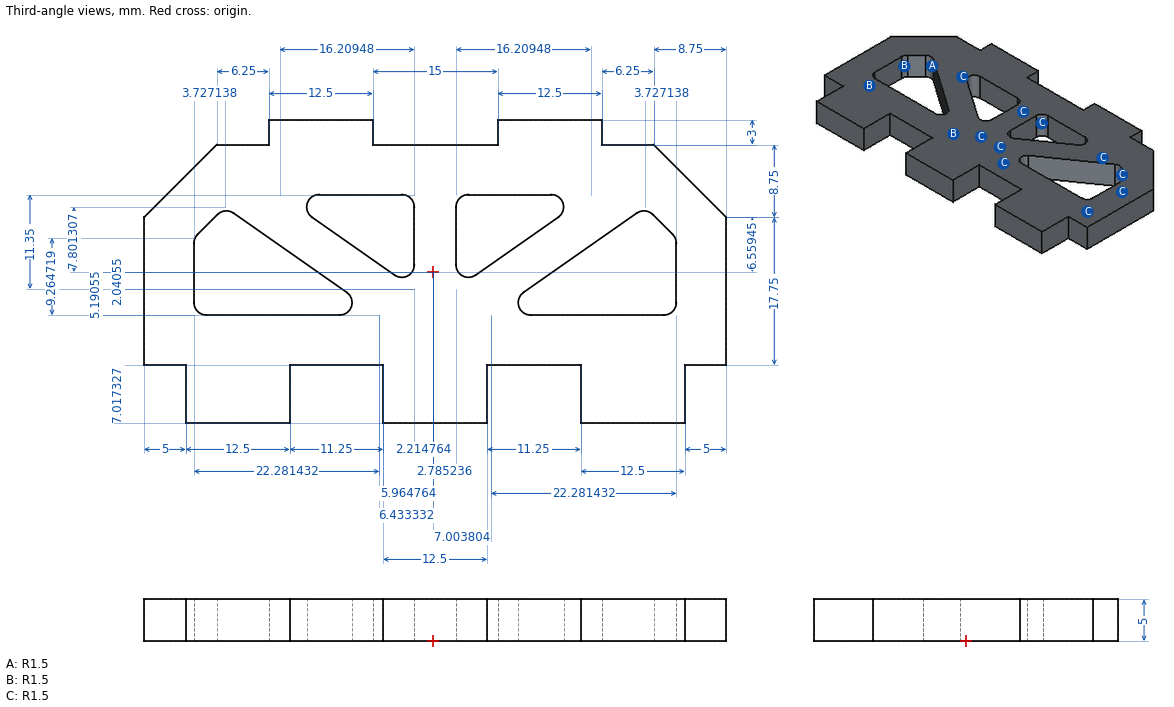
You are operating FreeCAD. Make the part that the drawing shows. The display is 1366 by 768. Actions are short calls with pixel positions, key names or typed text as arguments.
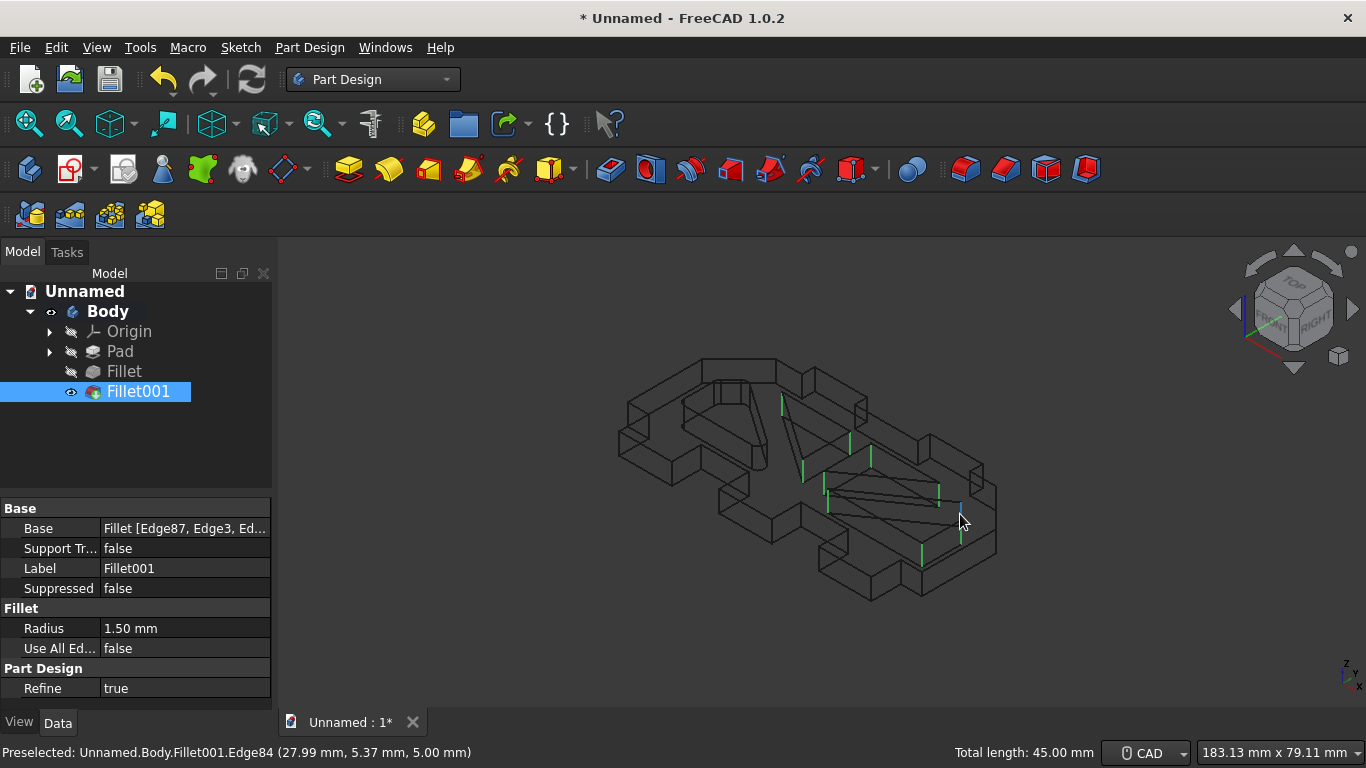
key(2)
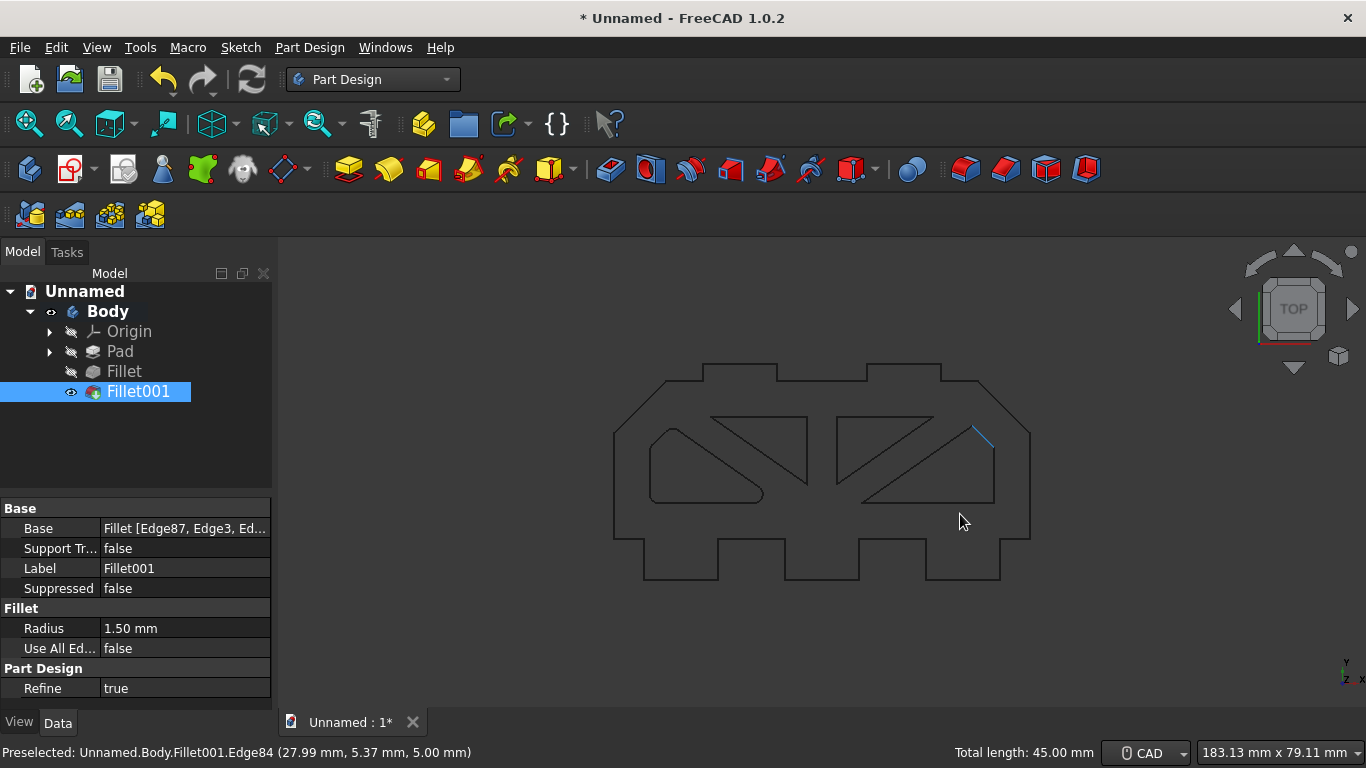
scroll(972, 425, up, 6)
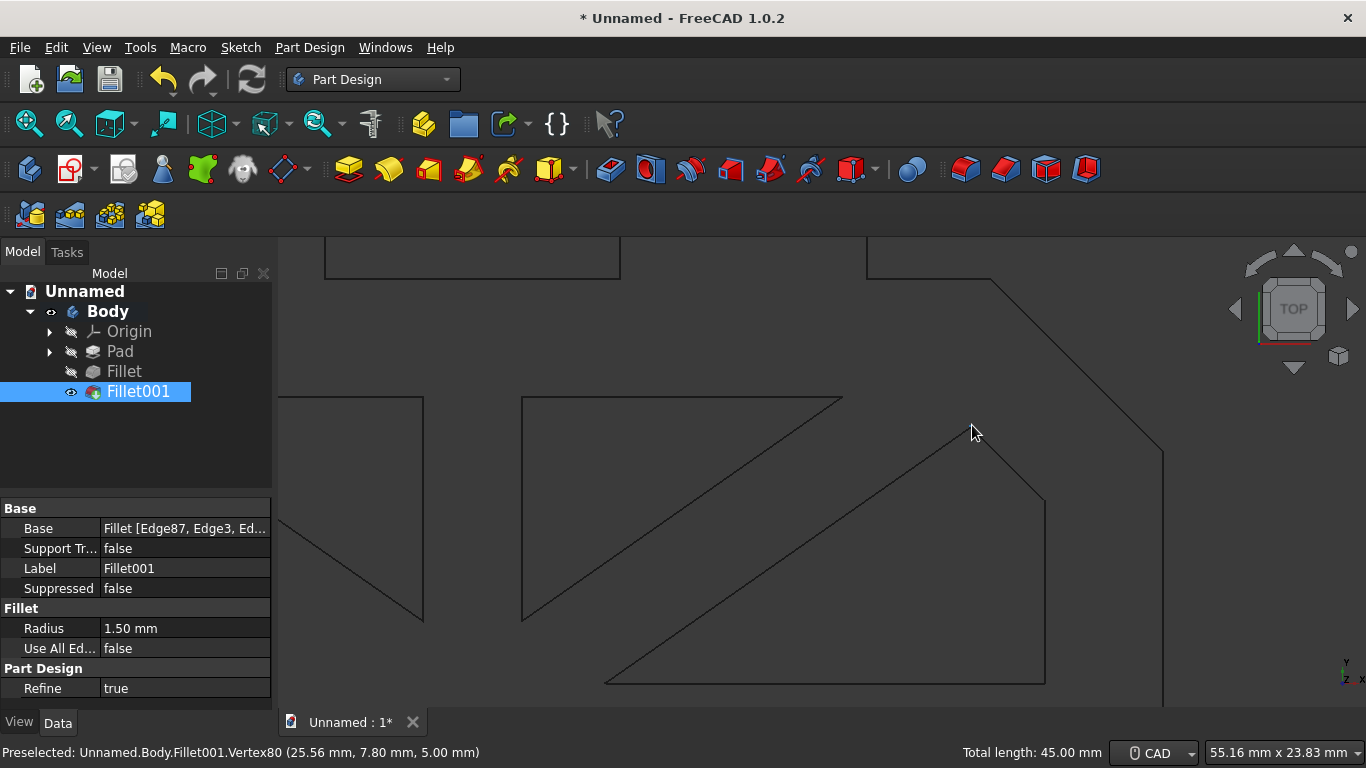
key(v)
key(f)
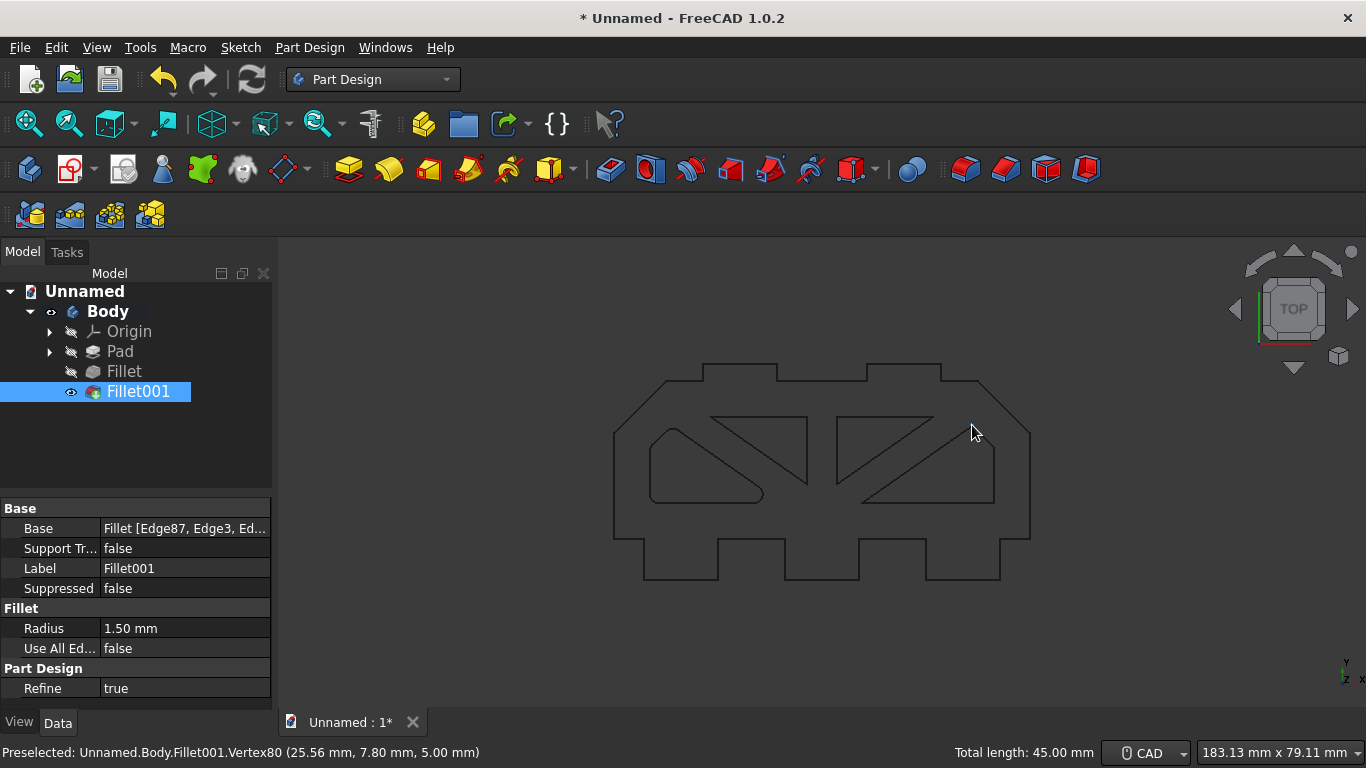
key(1)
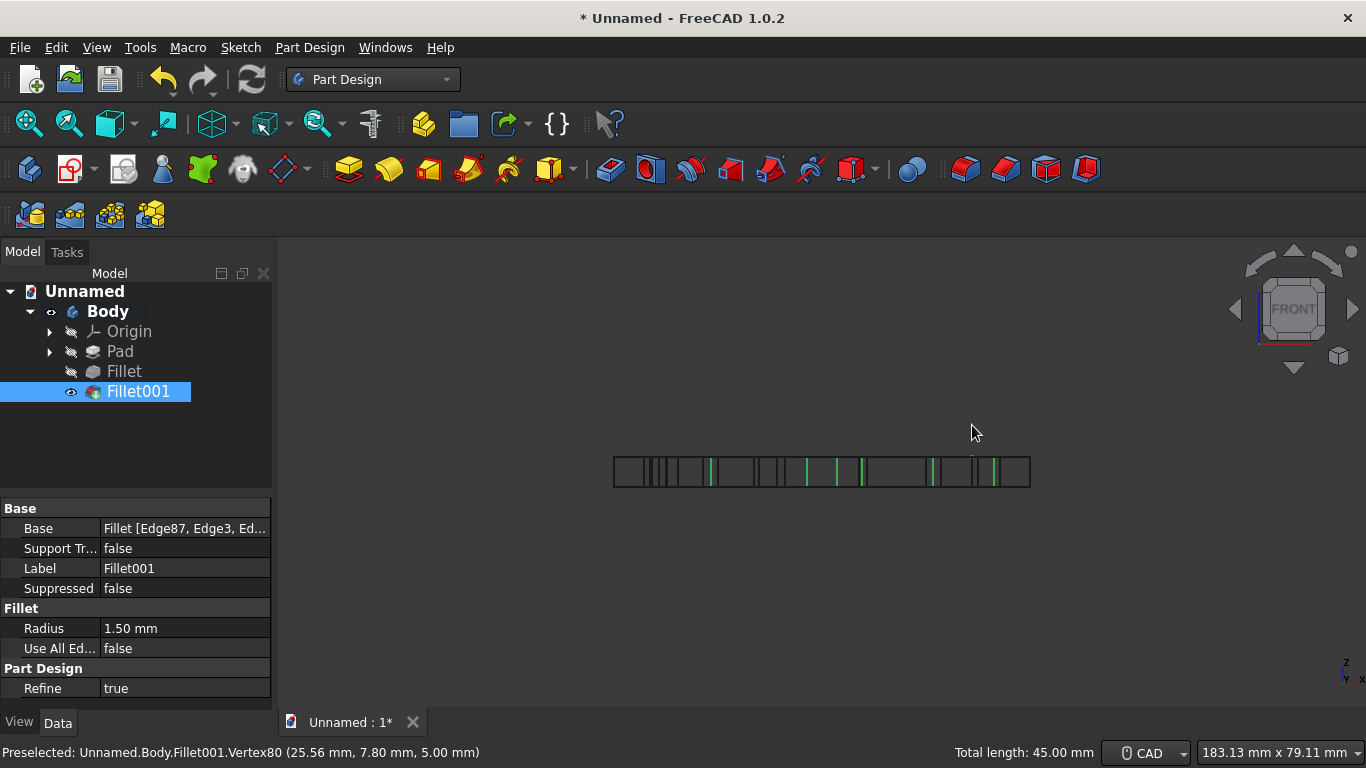
key(v)
key(f)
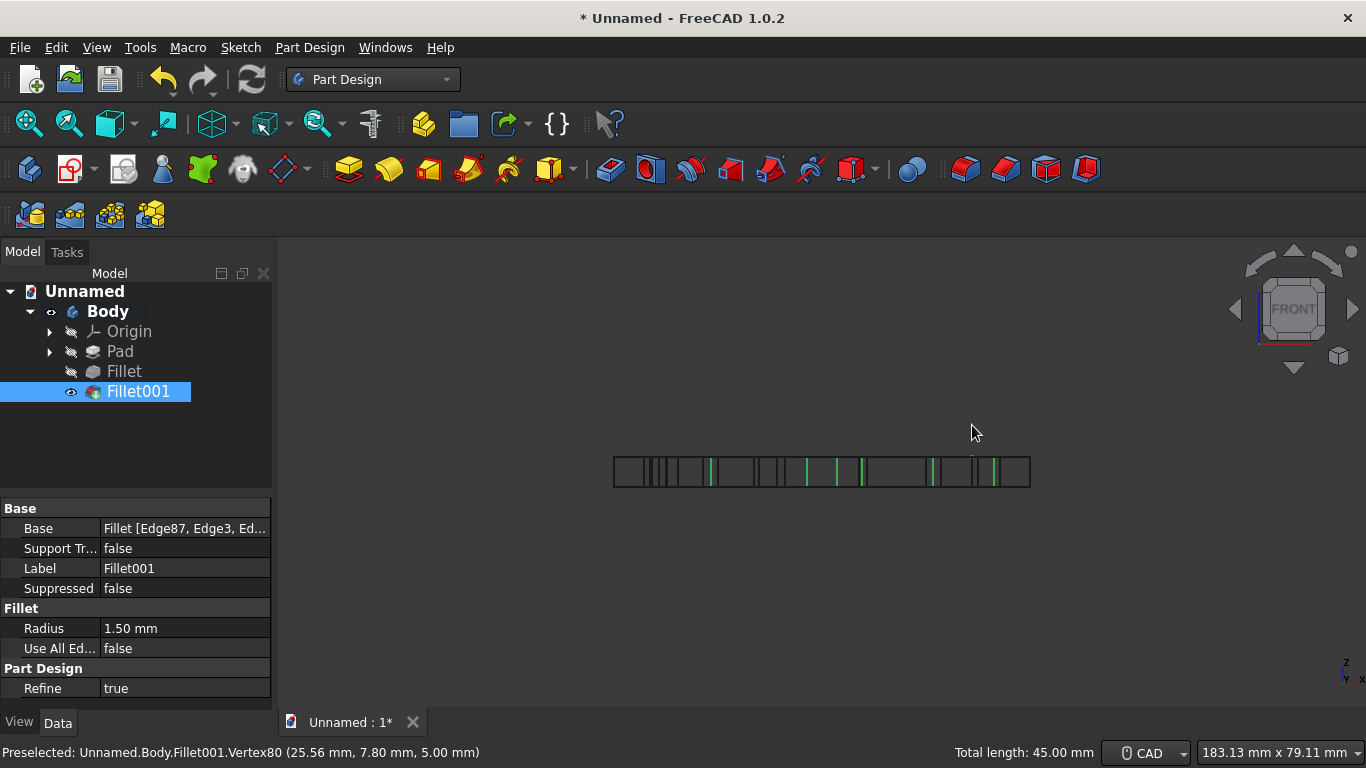
click(972, 471, ctrl)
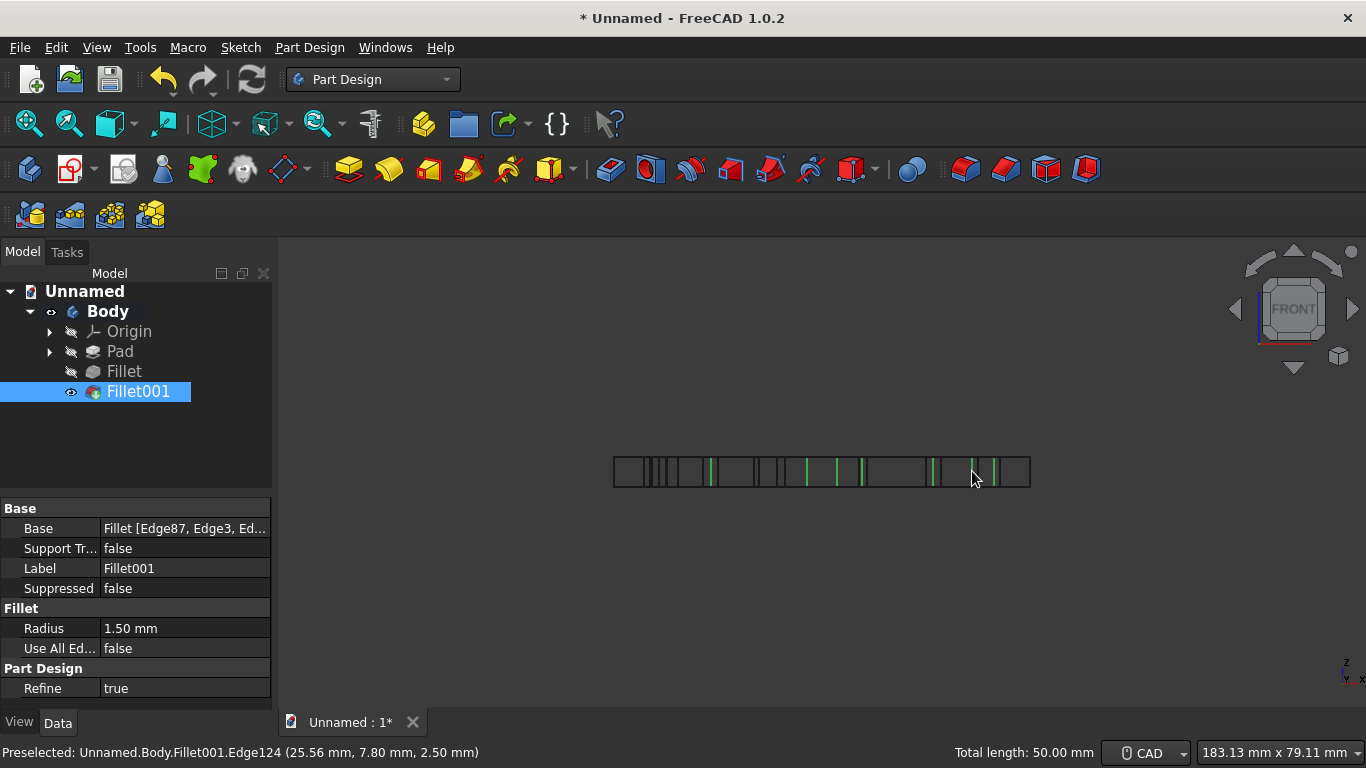
key(v)
key(1)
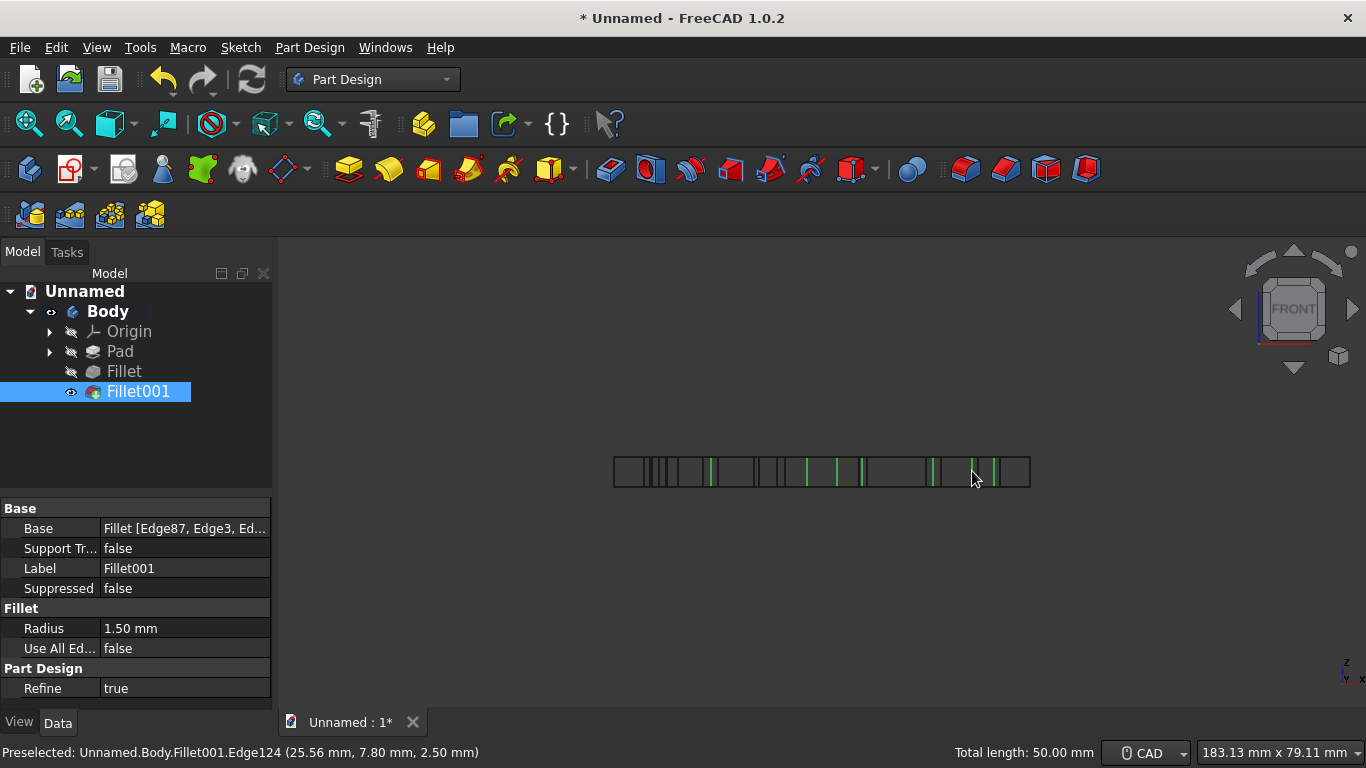
click(966, 170)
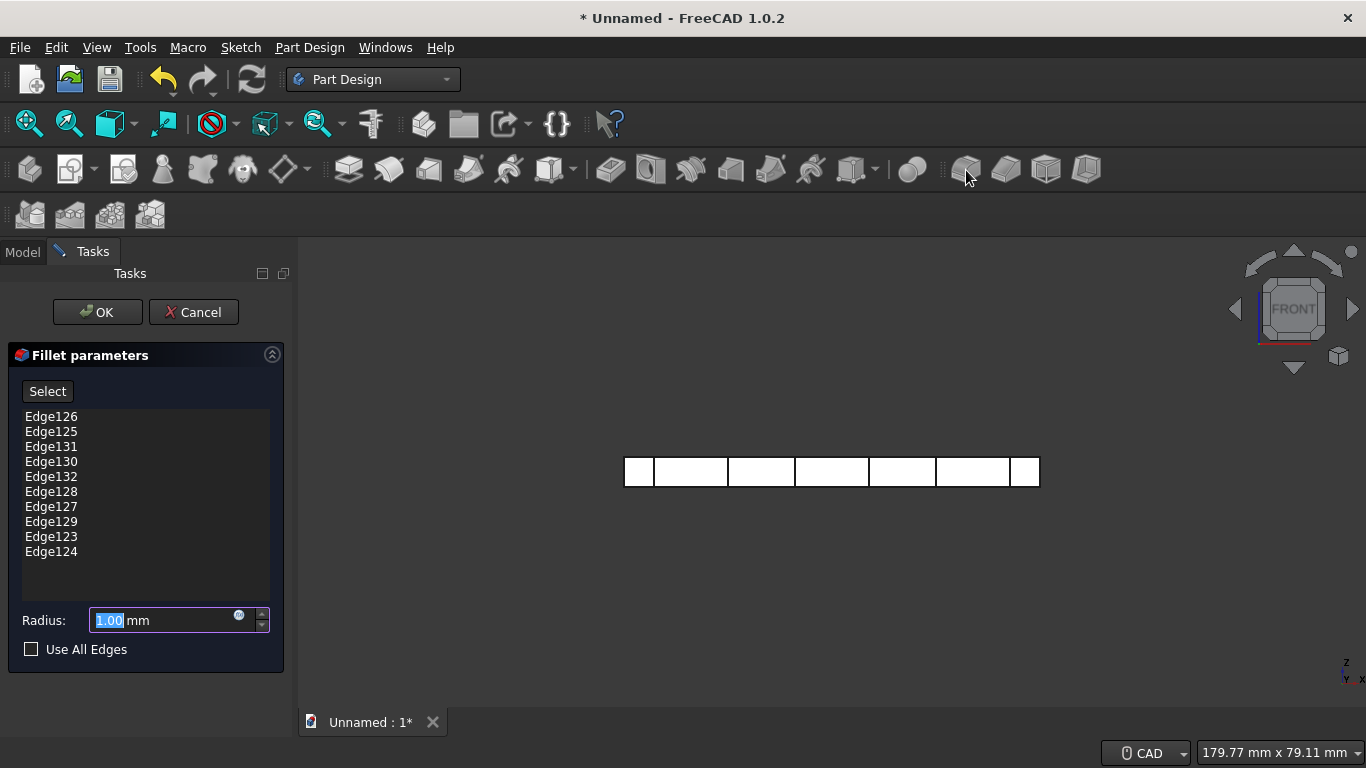
text(1.5)
key(Tab)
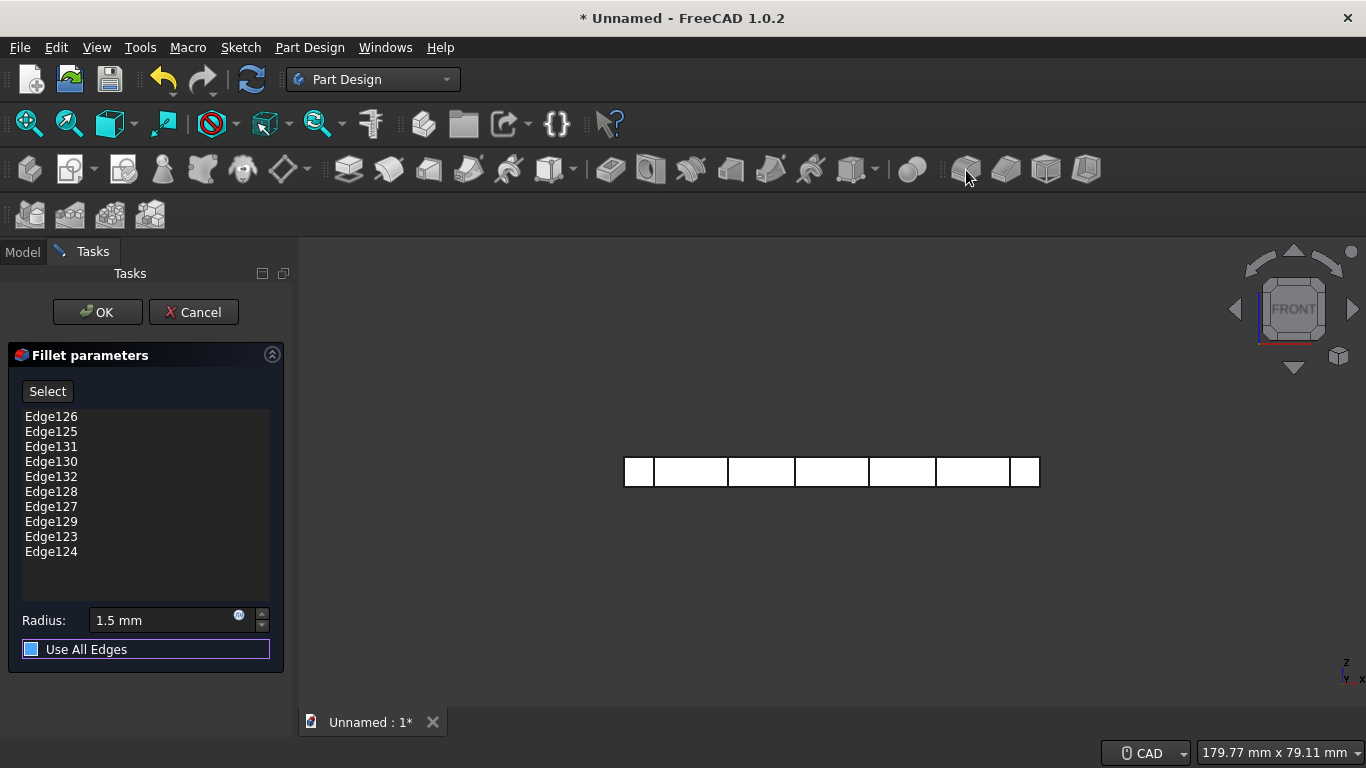
click(98, 312)